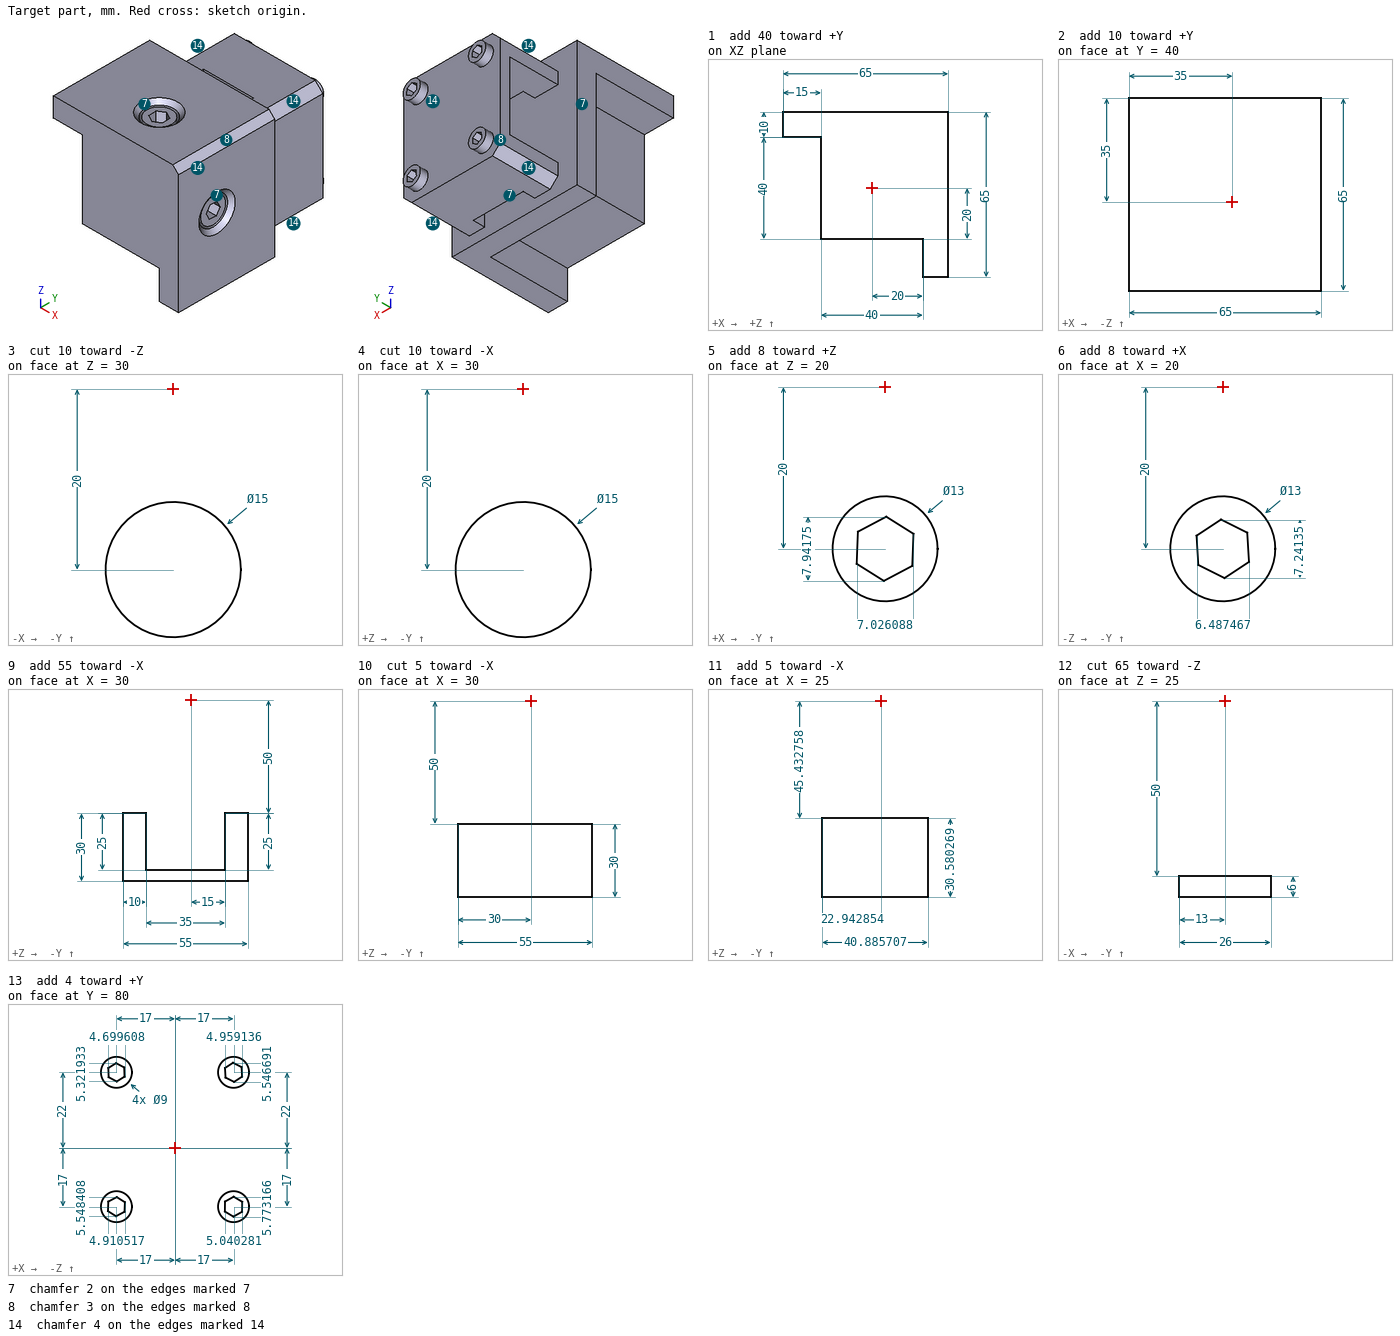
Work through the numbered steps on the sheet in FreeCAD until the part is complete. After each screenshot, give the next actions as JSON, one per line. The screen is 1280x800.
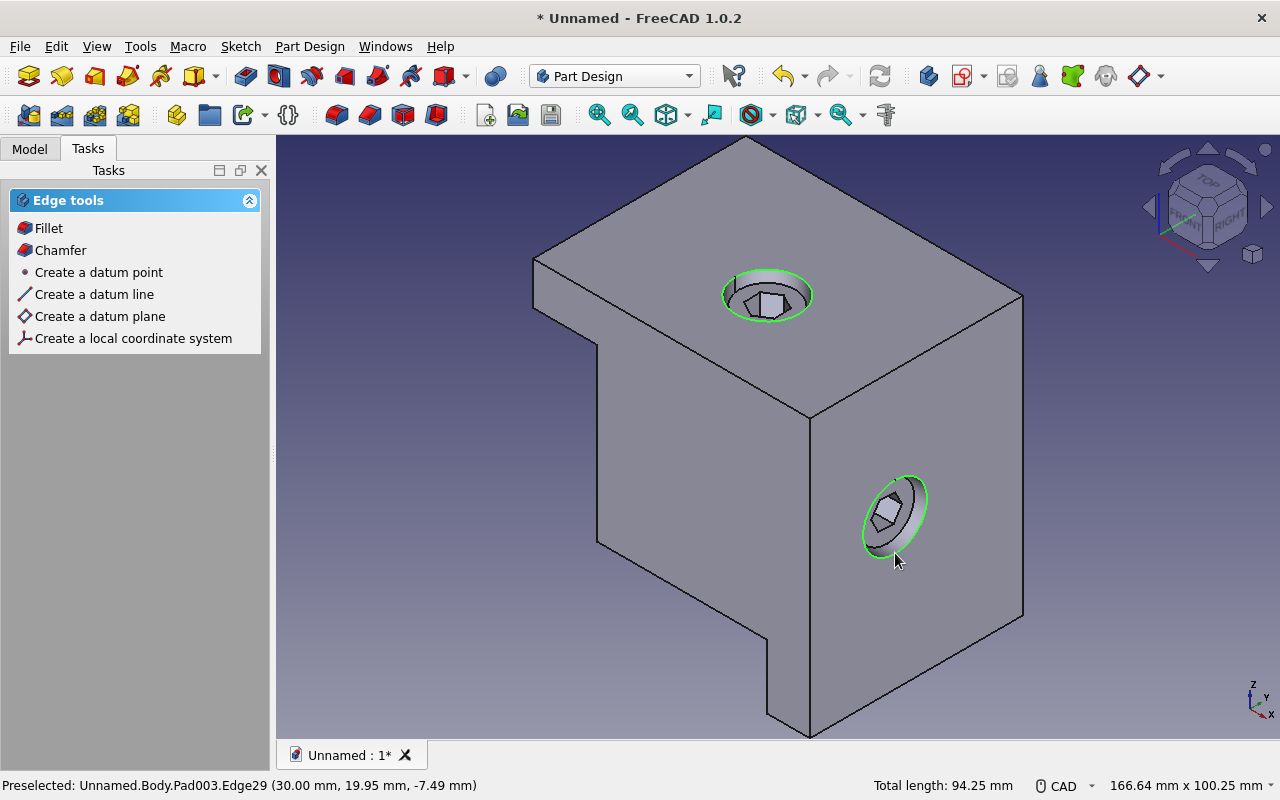
{"action": "left_click", "coordinate": [370, 116]}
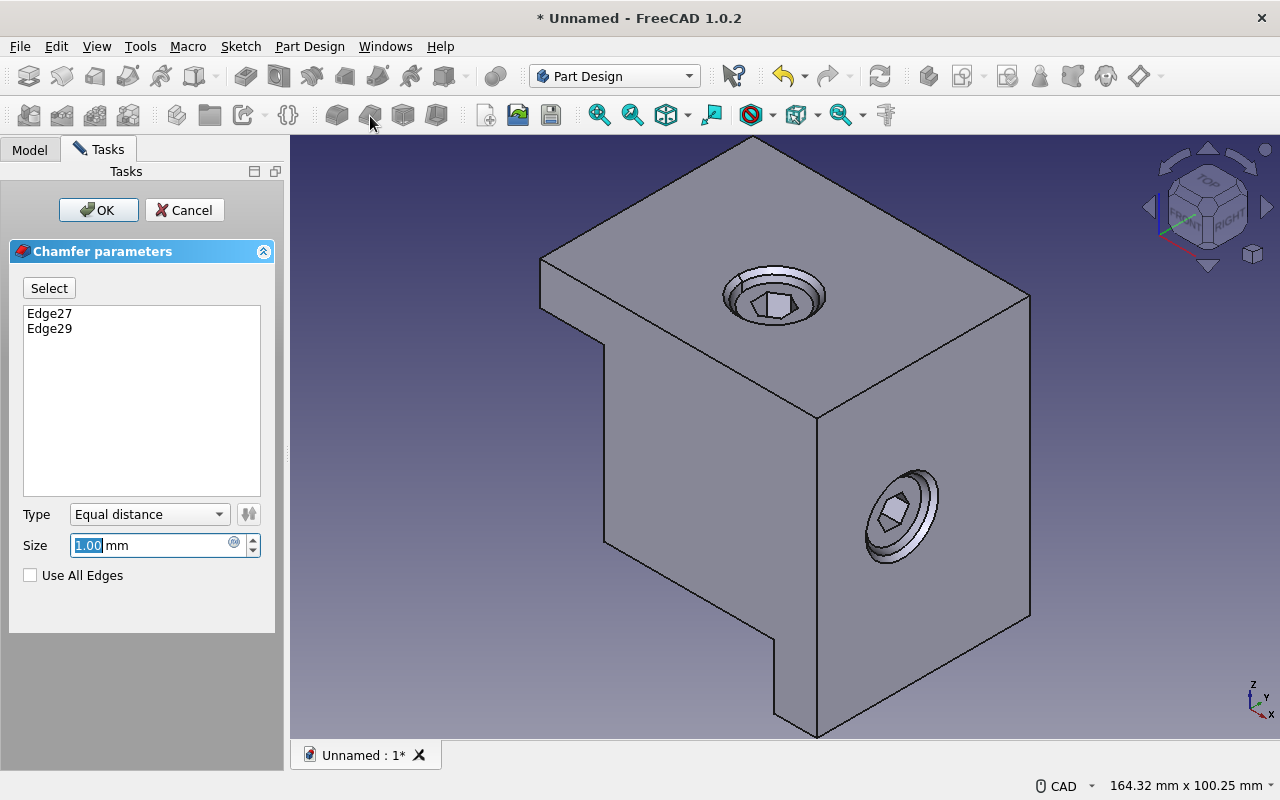
{"action": "type", "text": "2"}
{"action": "key", "text": "Tab"}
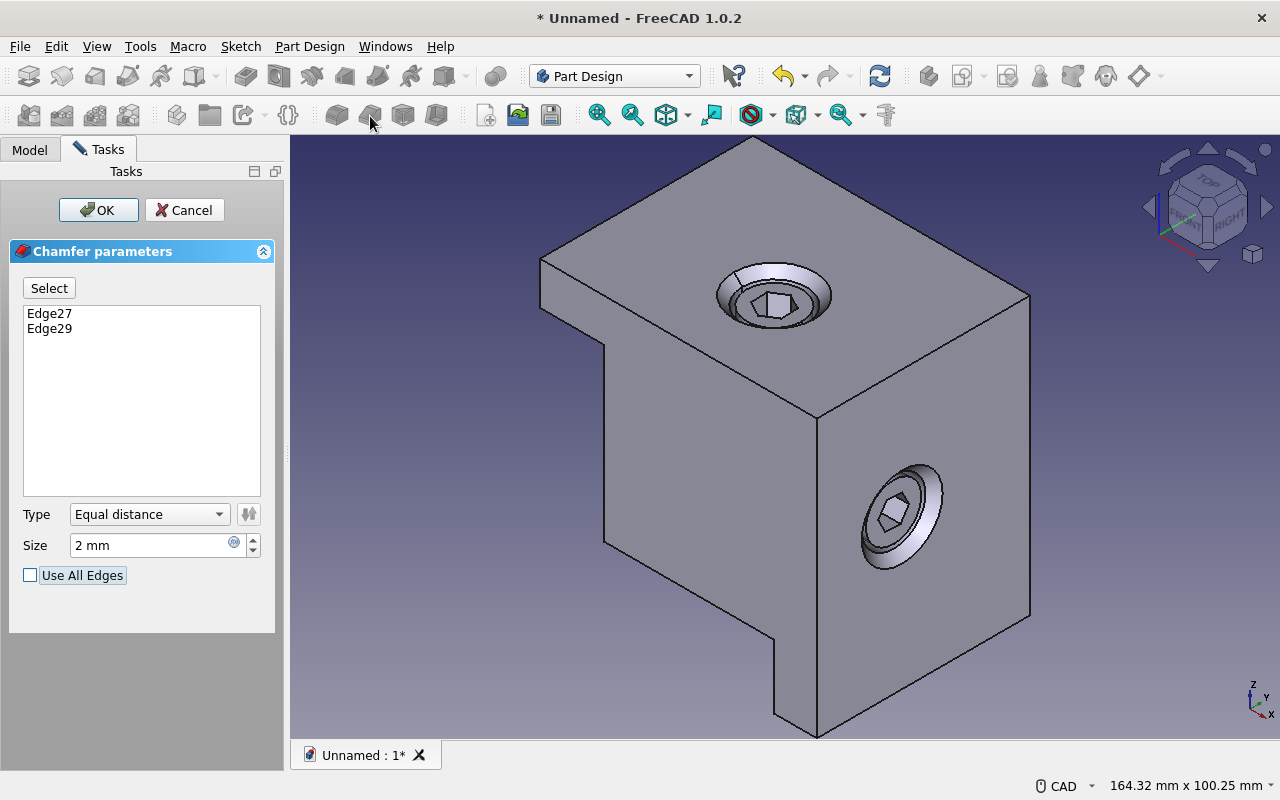
{"action": "left_click", "coordinate": [99, 210]}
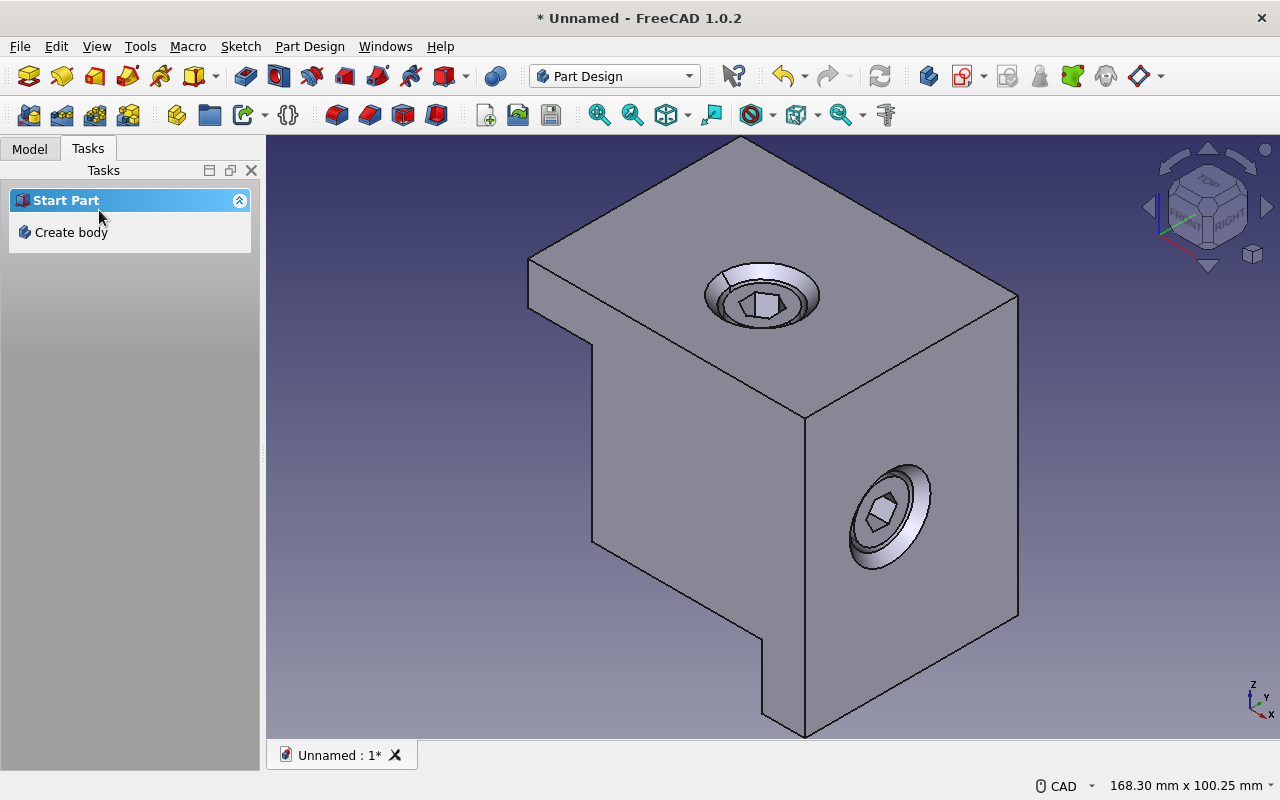
{"action": "left_click", "coordinate": [911, 356]}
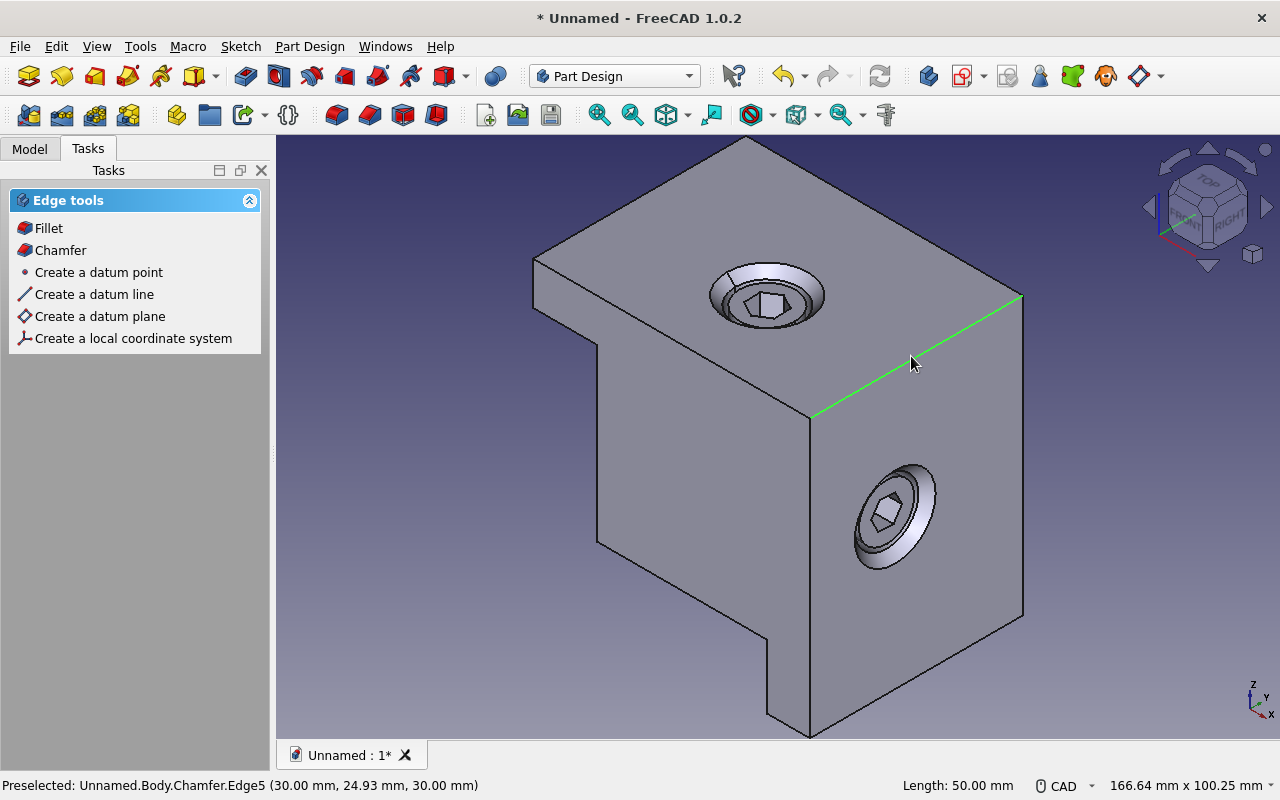
{"action": "left_click", "coordinate": [370, 116]}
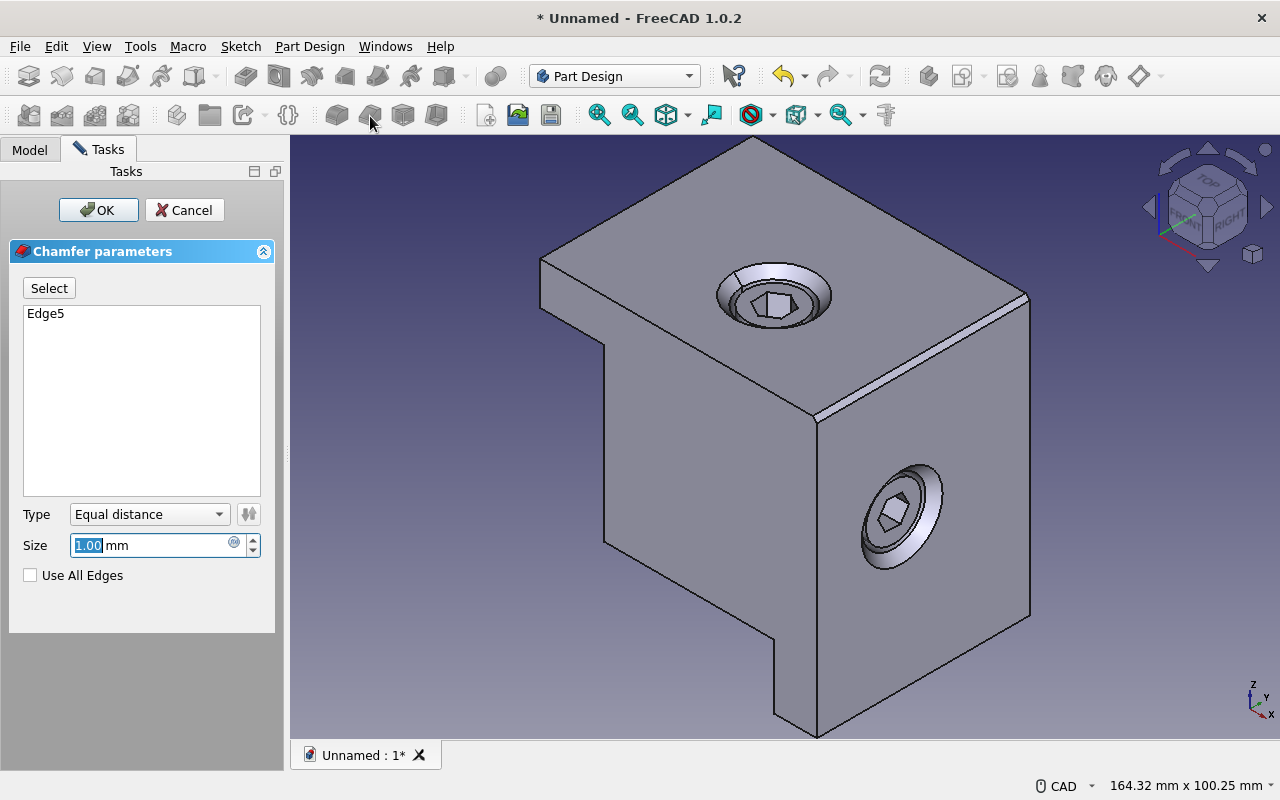
{"action": "type", "text": "3"}
{"action": "key", "text": "Tab"}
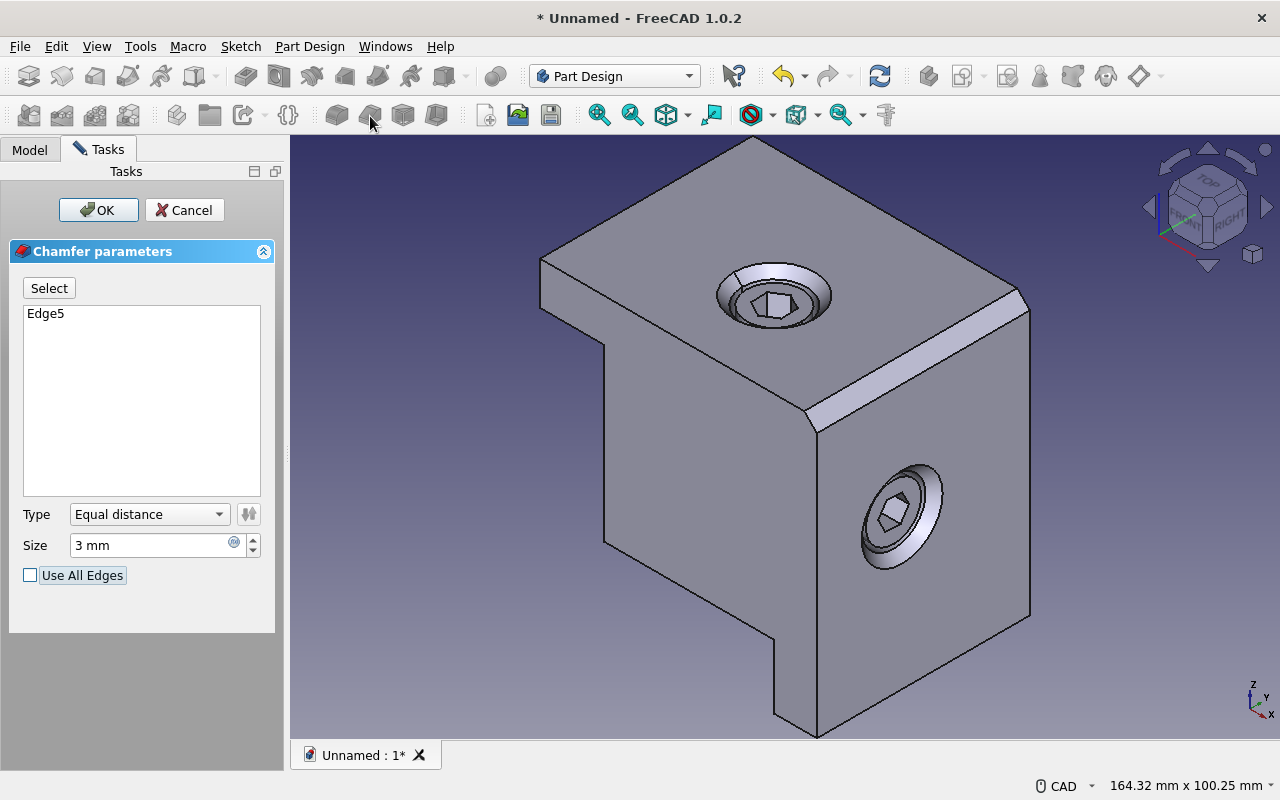
{"action": "left_click", "coordinate": [99, 210]}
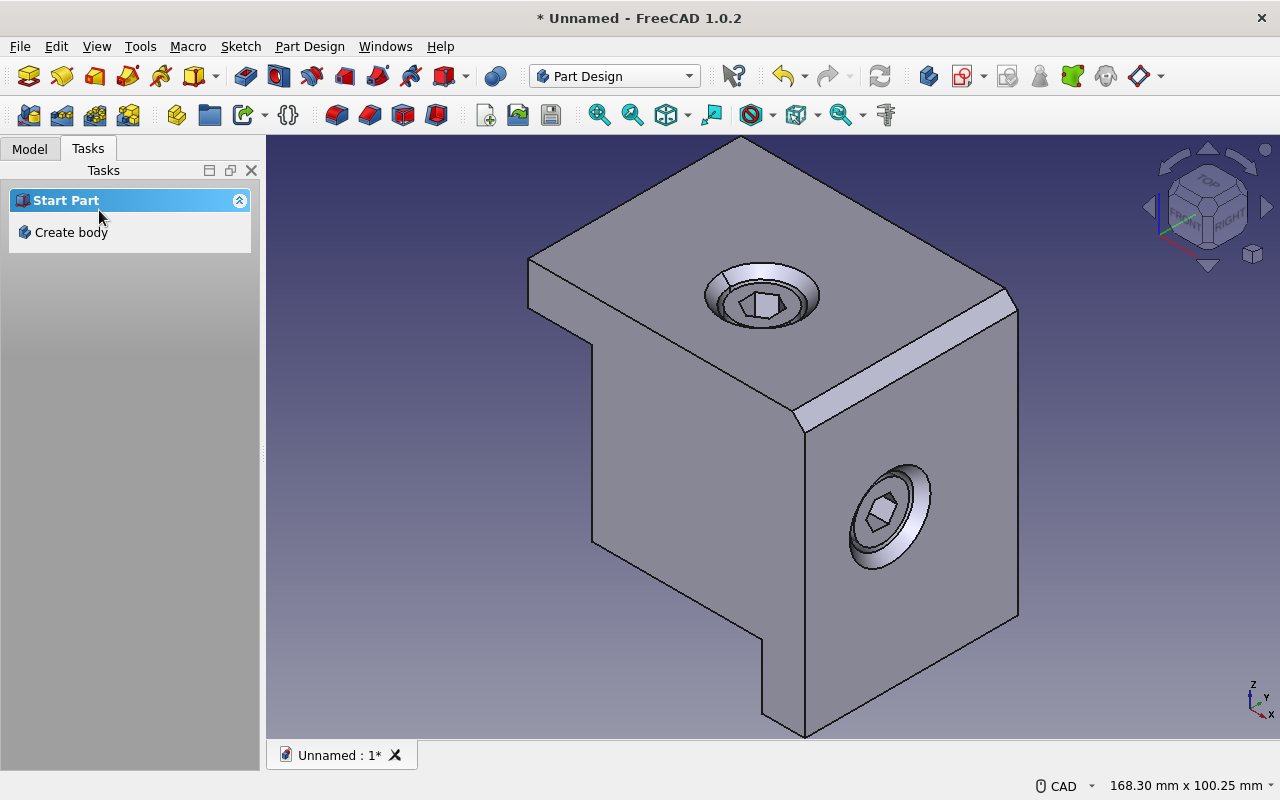
{"action": "left_click", "coordinate": [942, 593]}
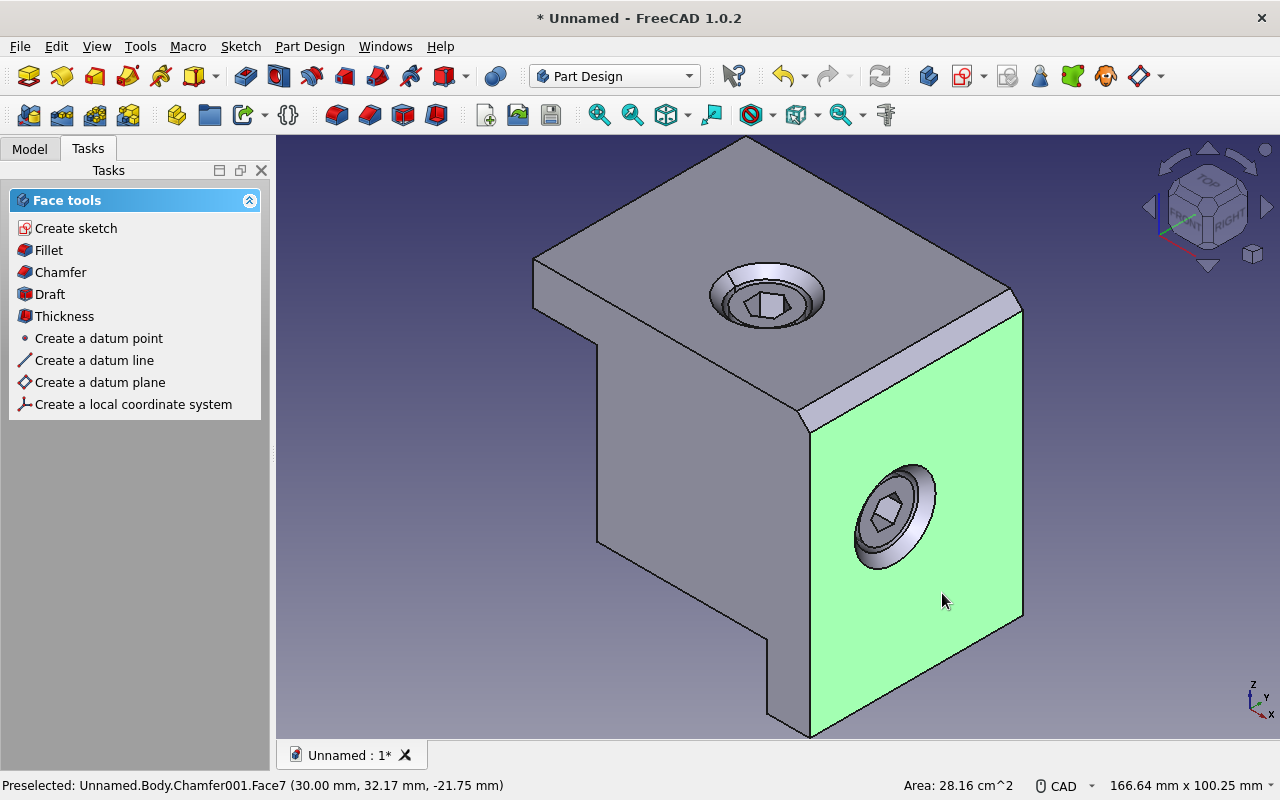
{"action": "left_click", "coordinate": [962, 76]}